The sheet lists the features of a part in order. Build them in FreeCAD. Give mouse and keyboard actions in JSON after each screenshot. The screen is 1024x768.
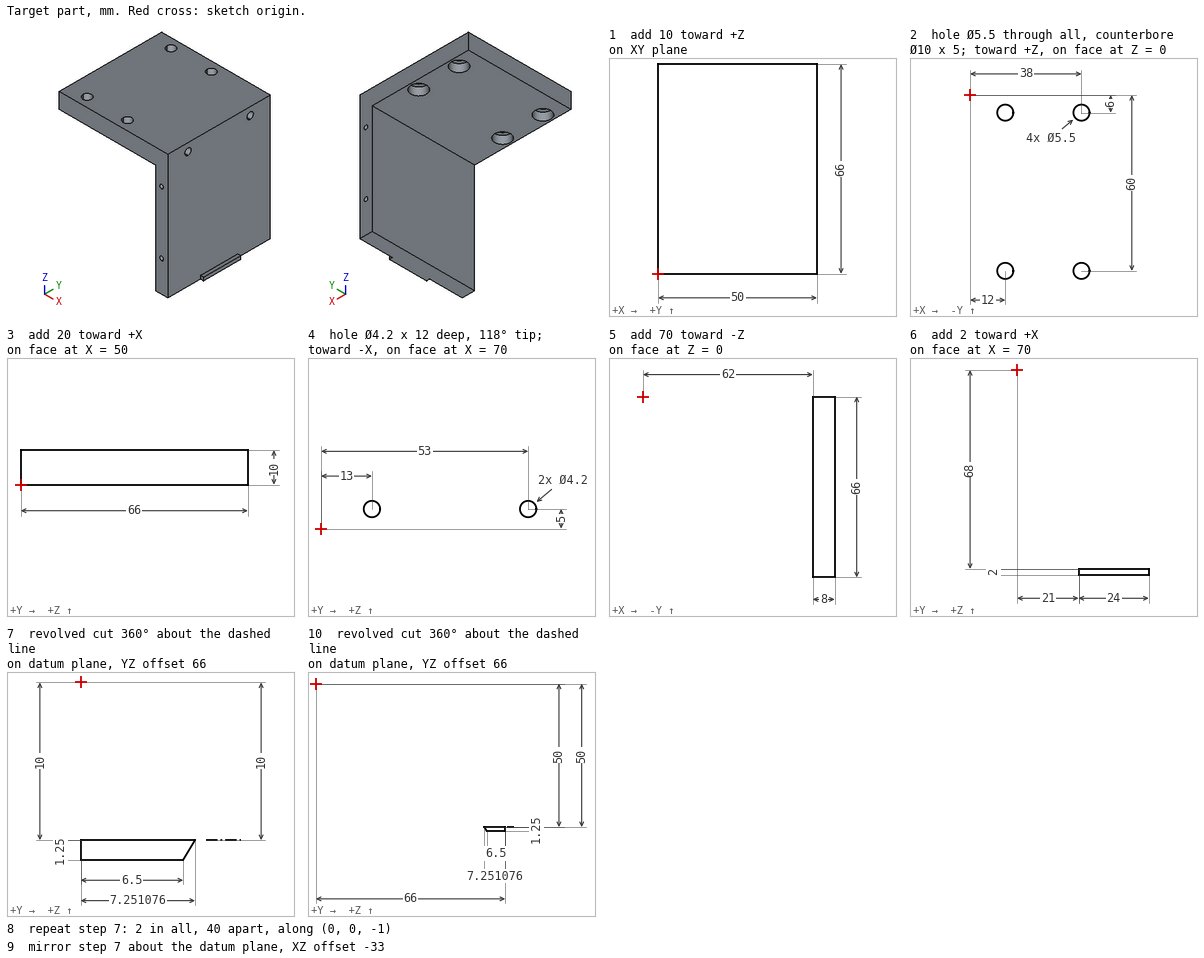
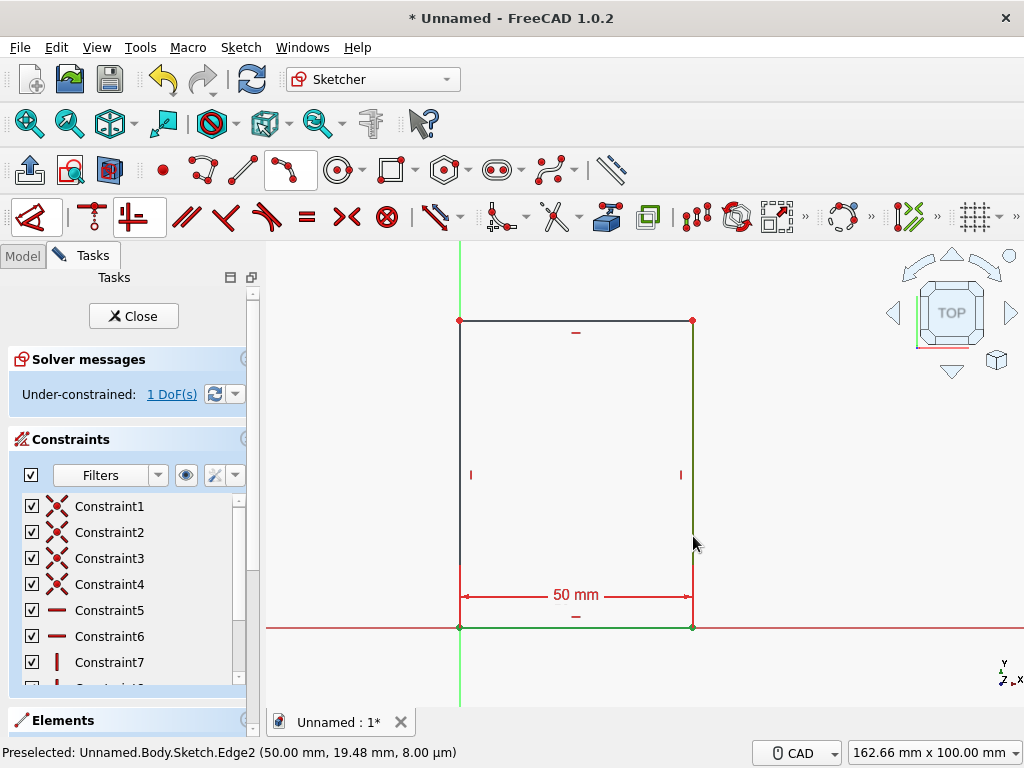
{"action": "key", "text": "i"}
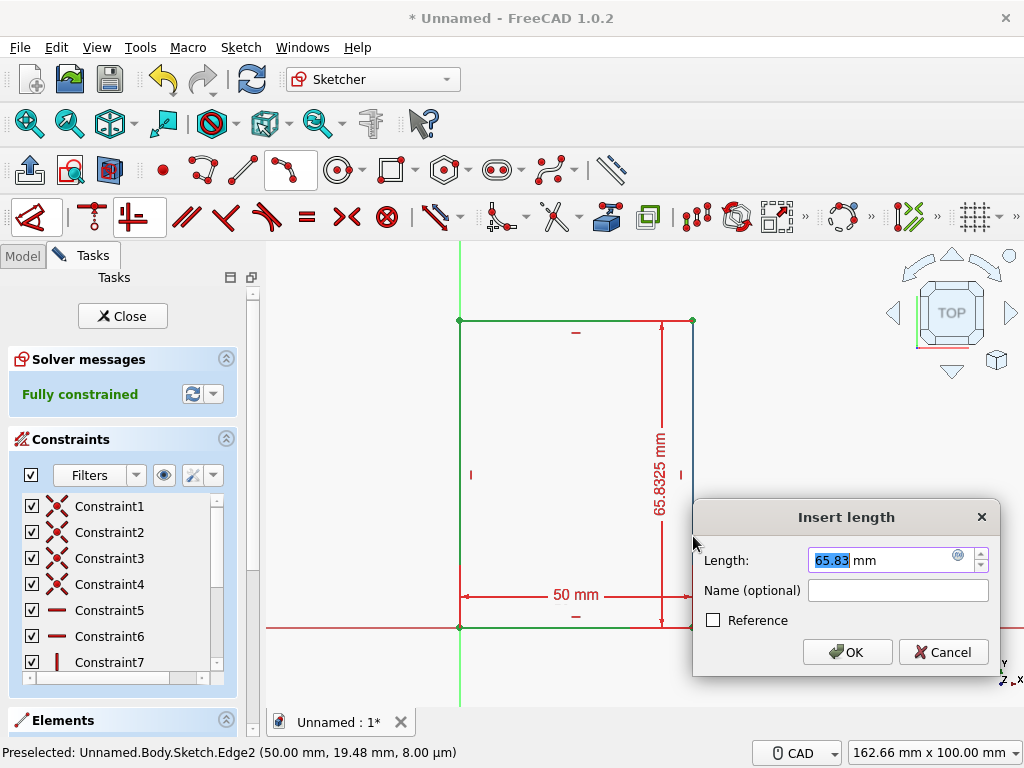
{"action": "type", "text": "66"}
{"action": "key", "text": "Return"}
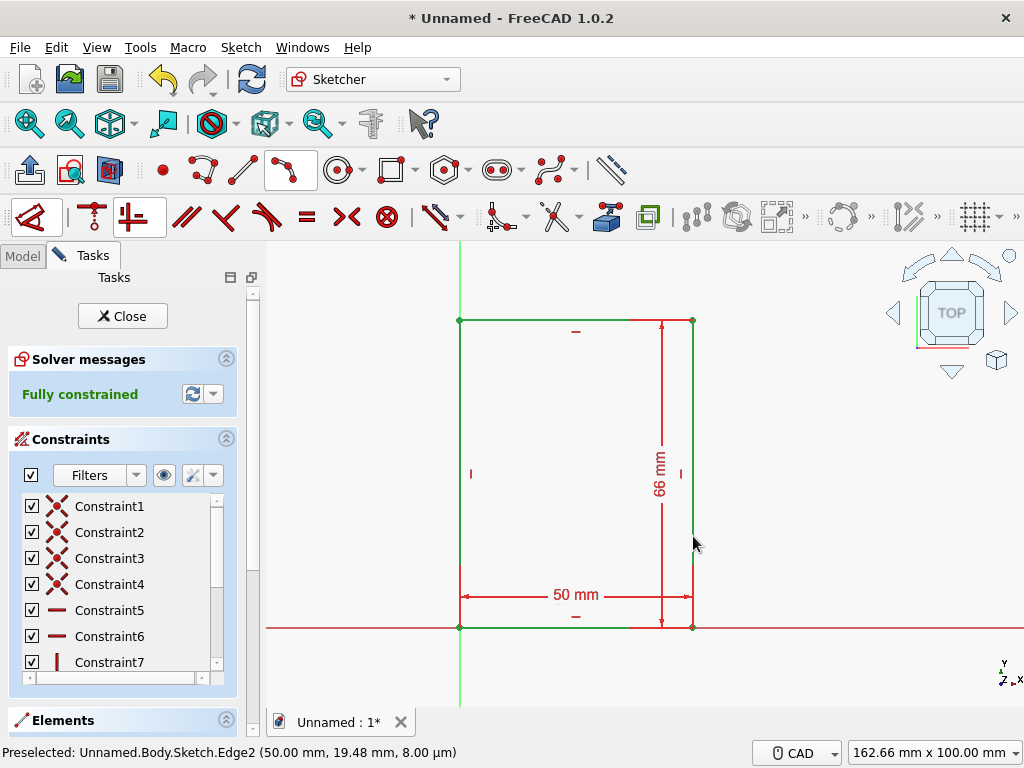
{"action": "left_click", "coordinate": [123, 316]}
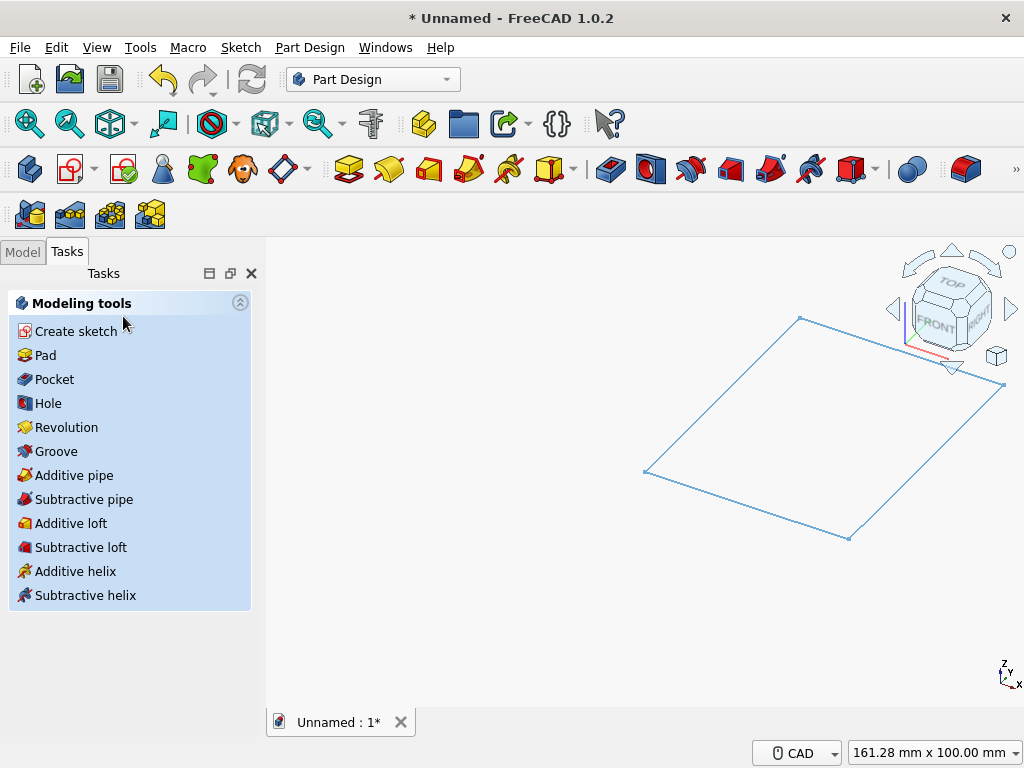
{"action": "left_click", "coordinate": [350, 170]}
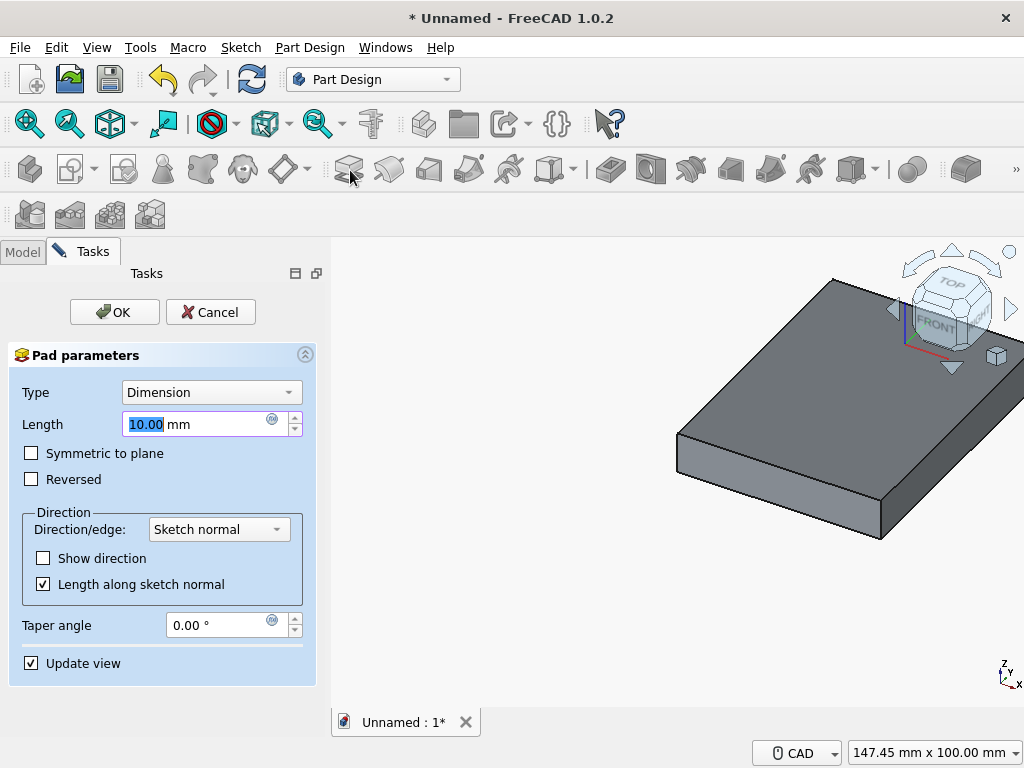
{"action": "type", "text": "10"}
{"action": "key", "text": "Tab"}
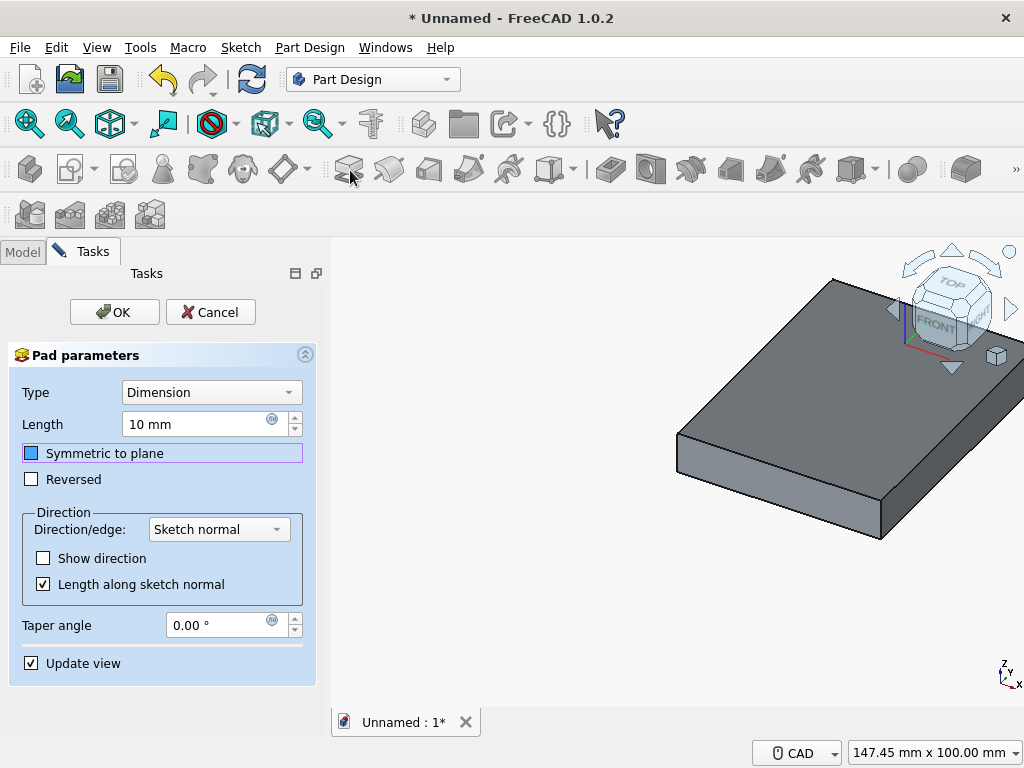
{"action": "left_click", "coordinate": [115, 312]}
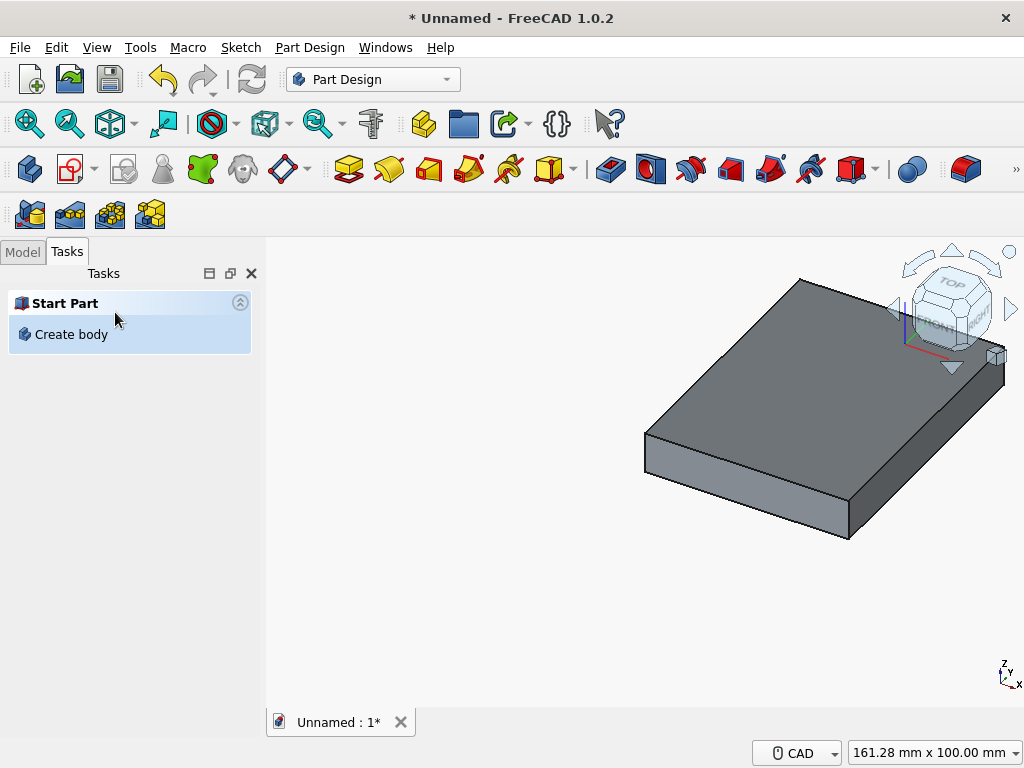
{"action": "key", "text": "5"}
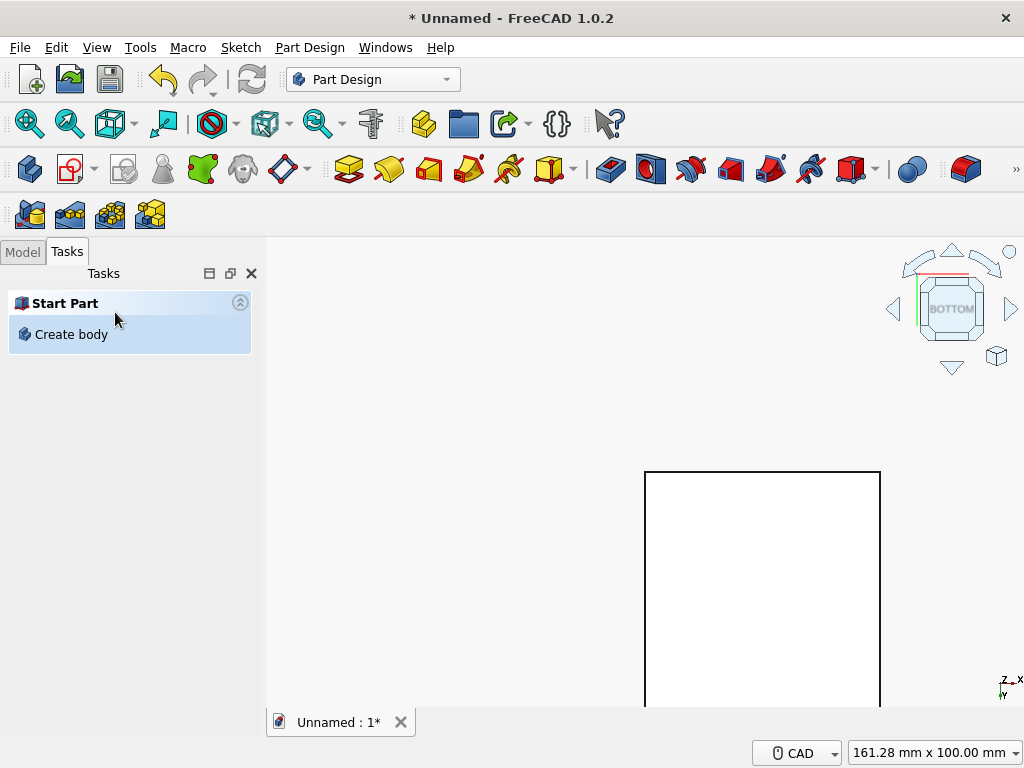
{"action": "left_click", "coordinate": [30, 124]}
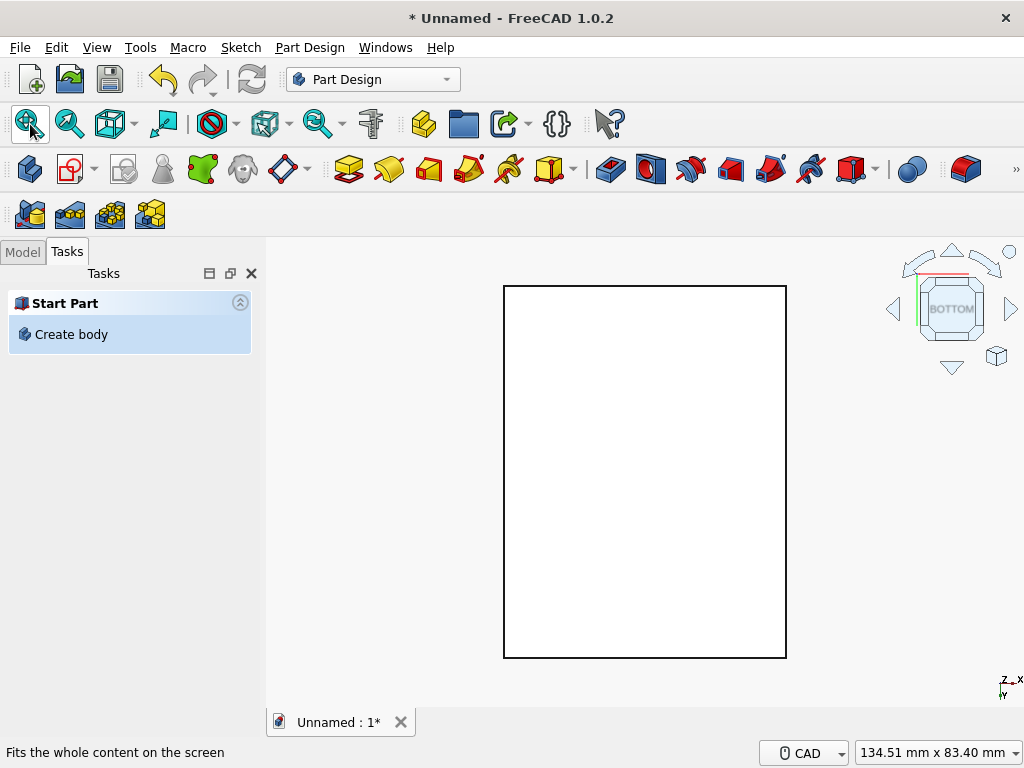
{"action": "left_click", "coordinate": [645, 471]}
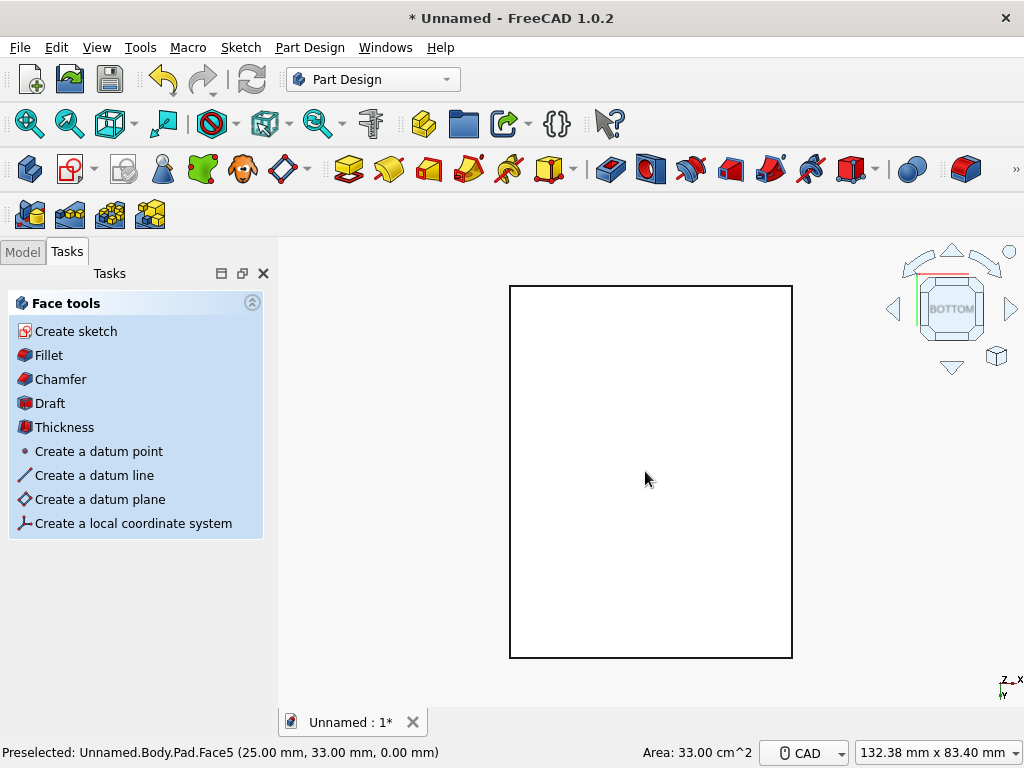
{"action": "left_click", "coordinate": [70, 170]}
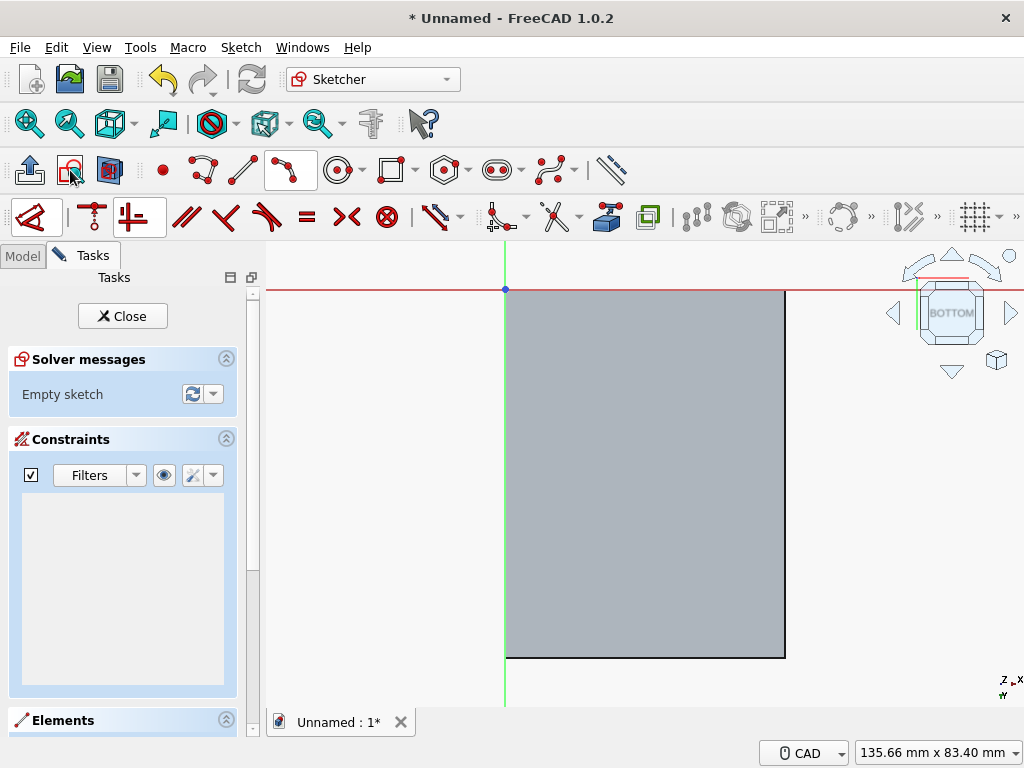
{"action": "scroll", "coordinate": [384, 515], "scroll_direction": "down", "scroll_amount": 1}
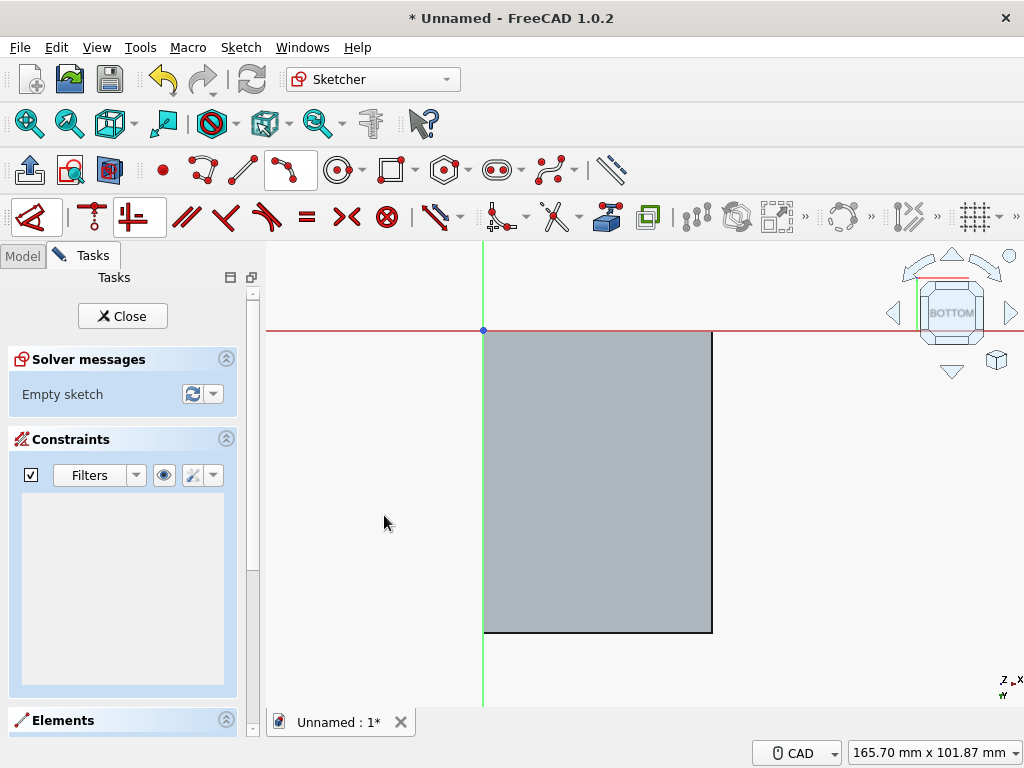
{"action": "key", "text": "g c"}